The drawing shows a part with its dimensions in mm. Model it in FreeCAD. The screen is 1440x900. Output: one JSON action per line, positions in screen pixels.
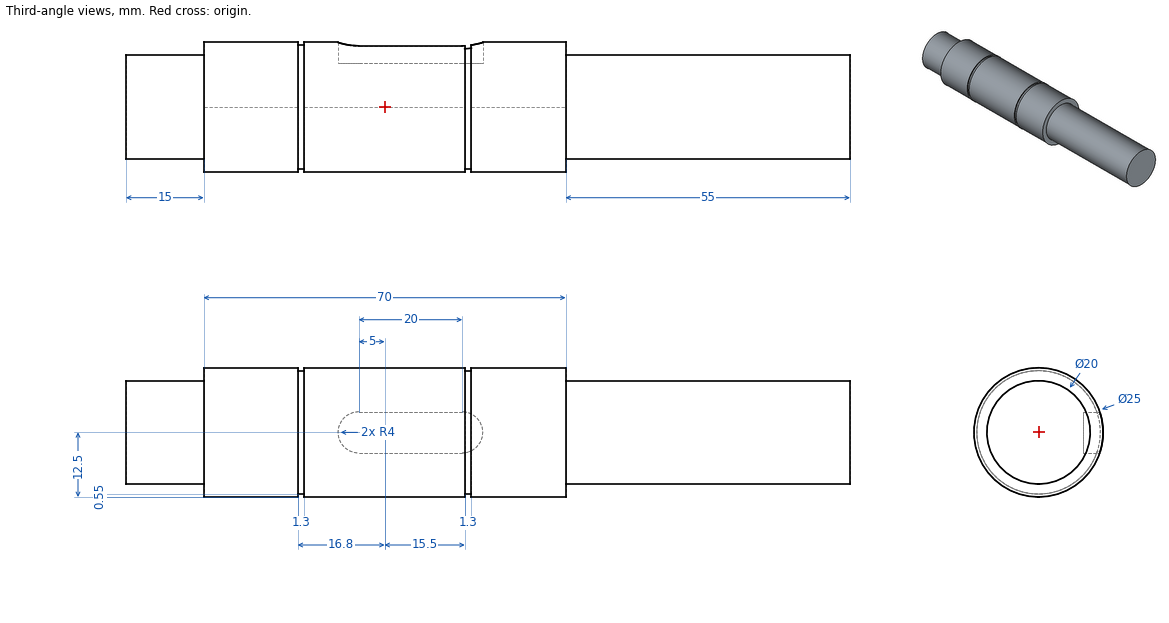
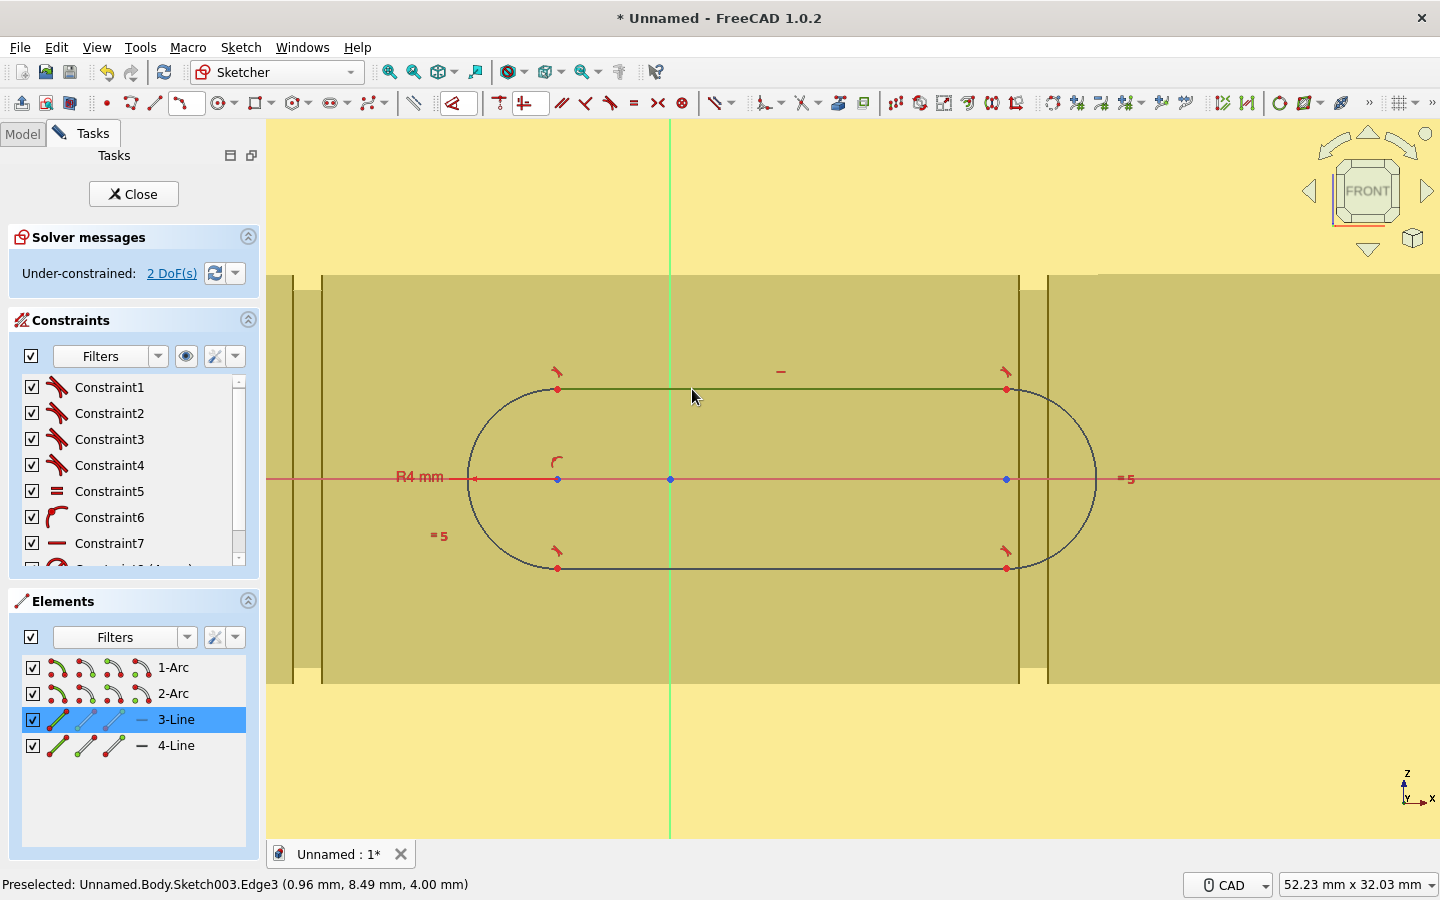
{"action": "key", "text": "l"}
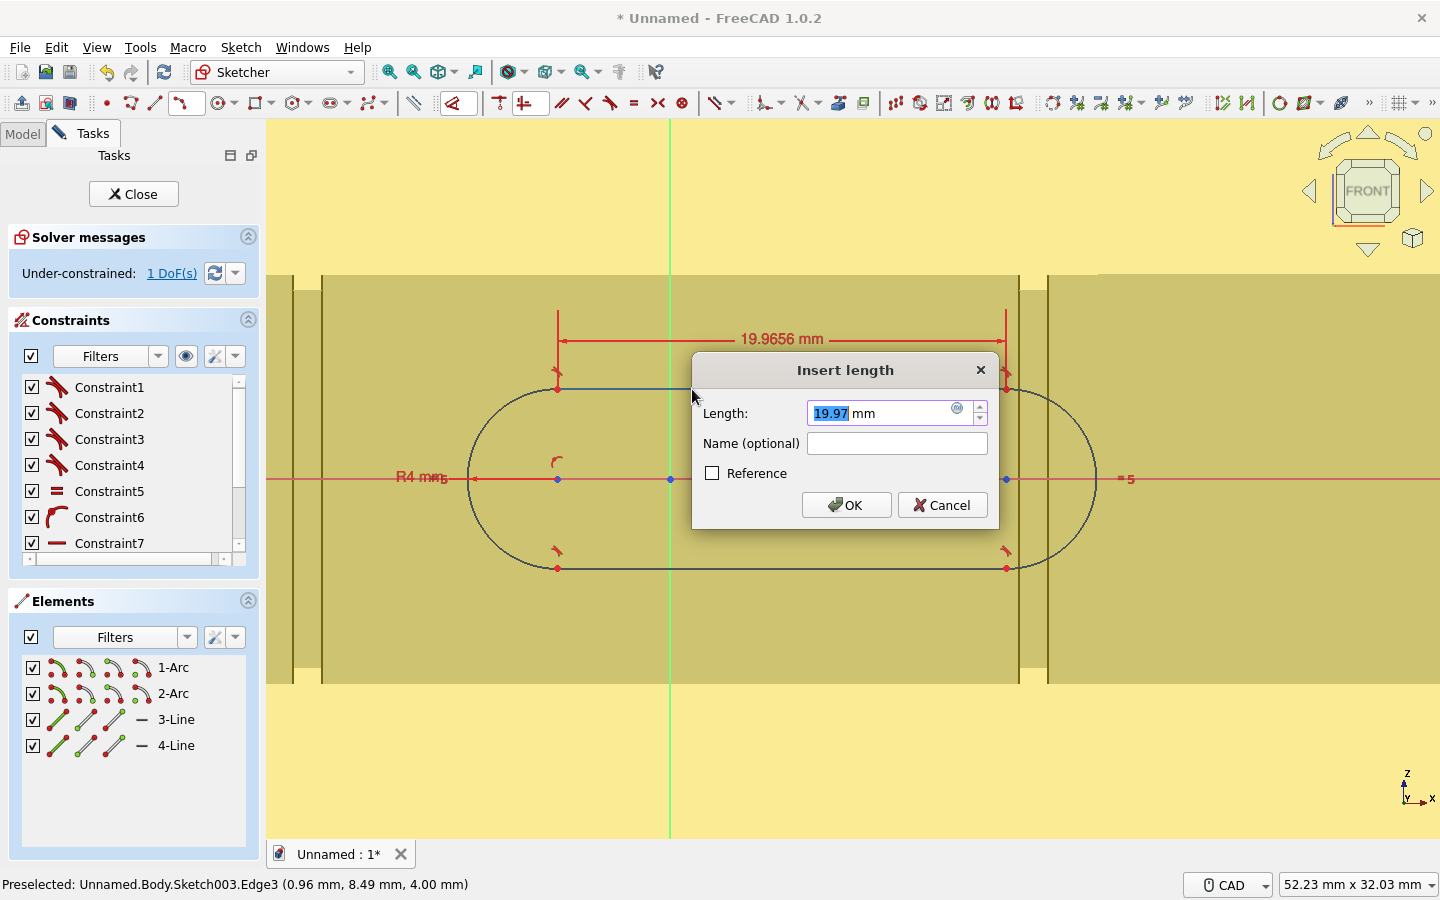
{"action": "type", "text": "20"}
{"action": "key", "text": "Return"}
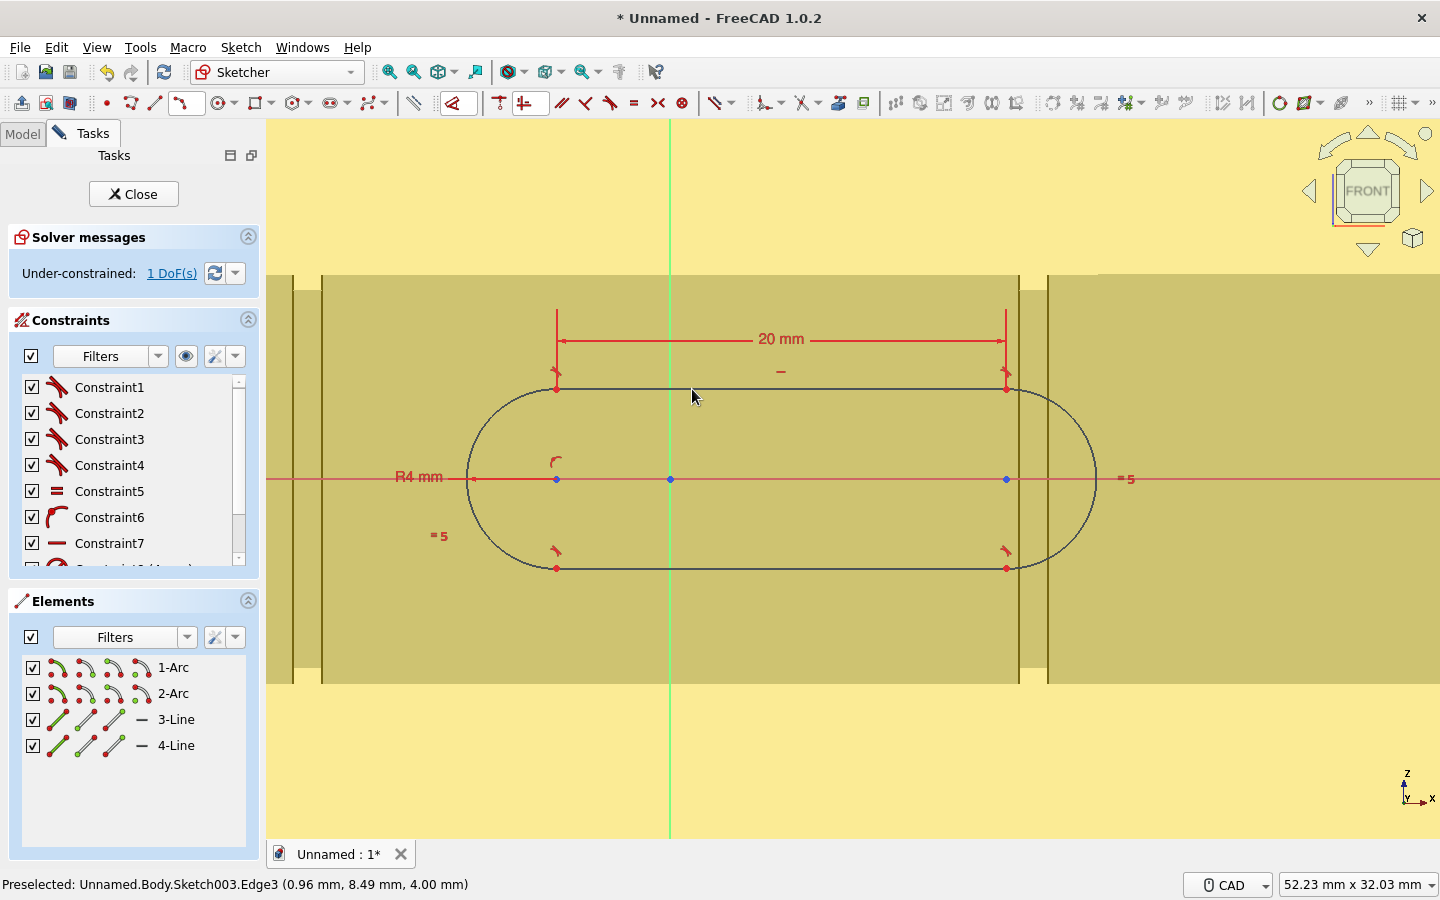
{"action": "left_click", "coordinate": [557, 389]}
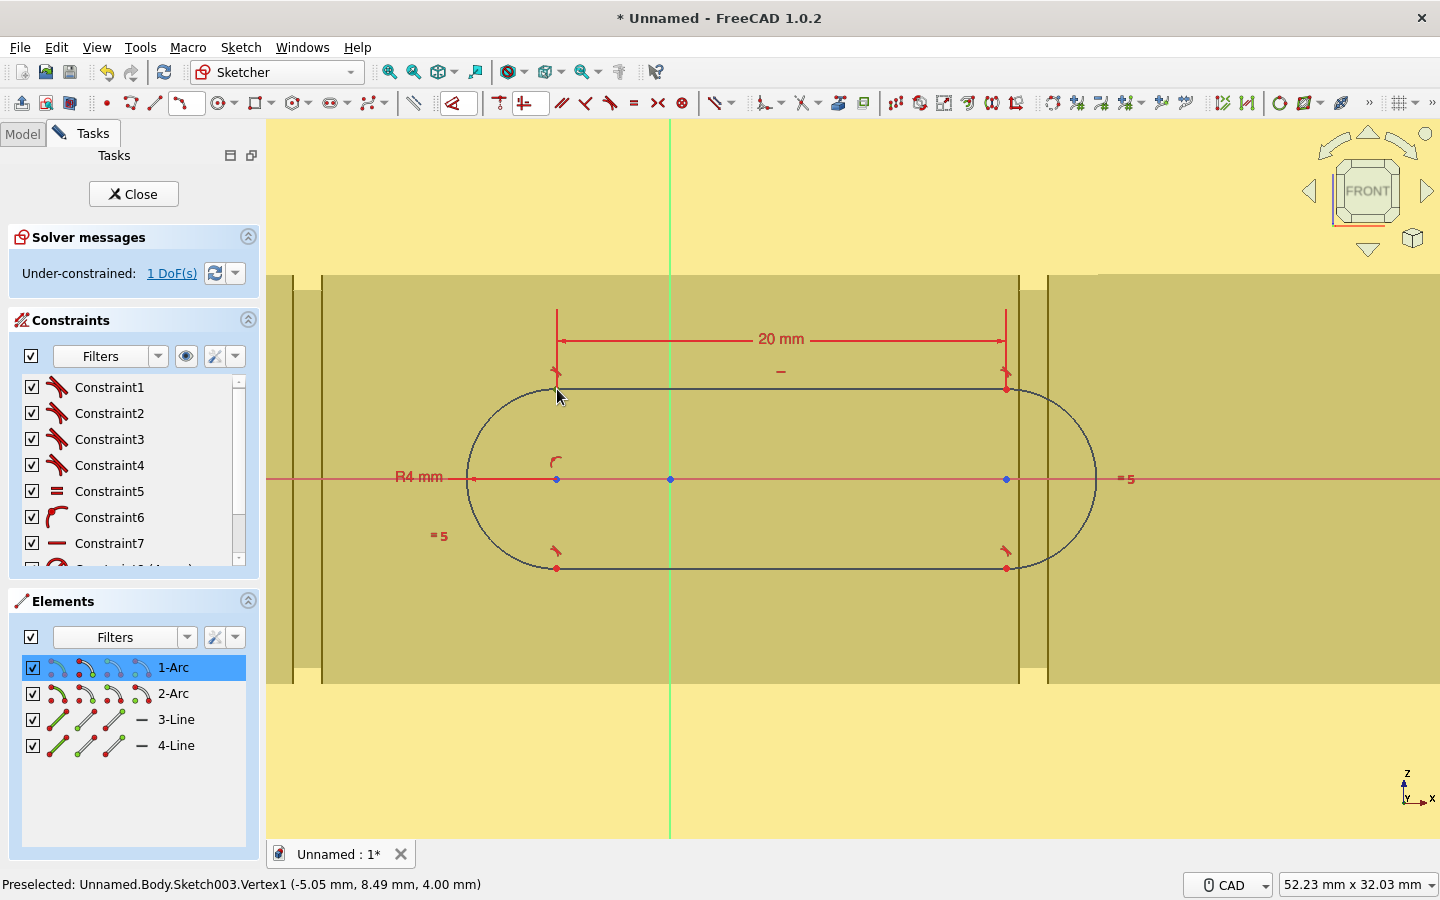
{"action": "left_click", "coordinate": [472, 104]}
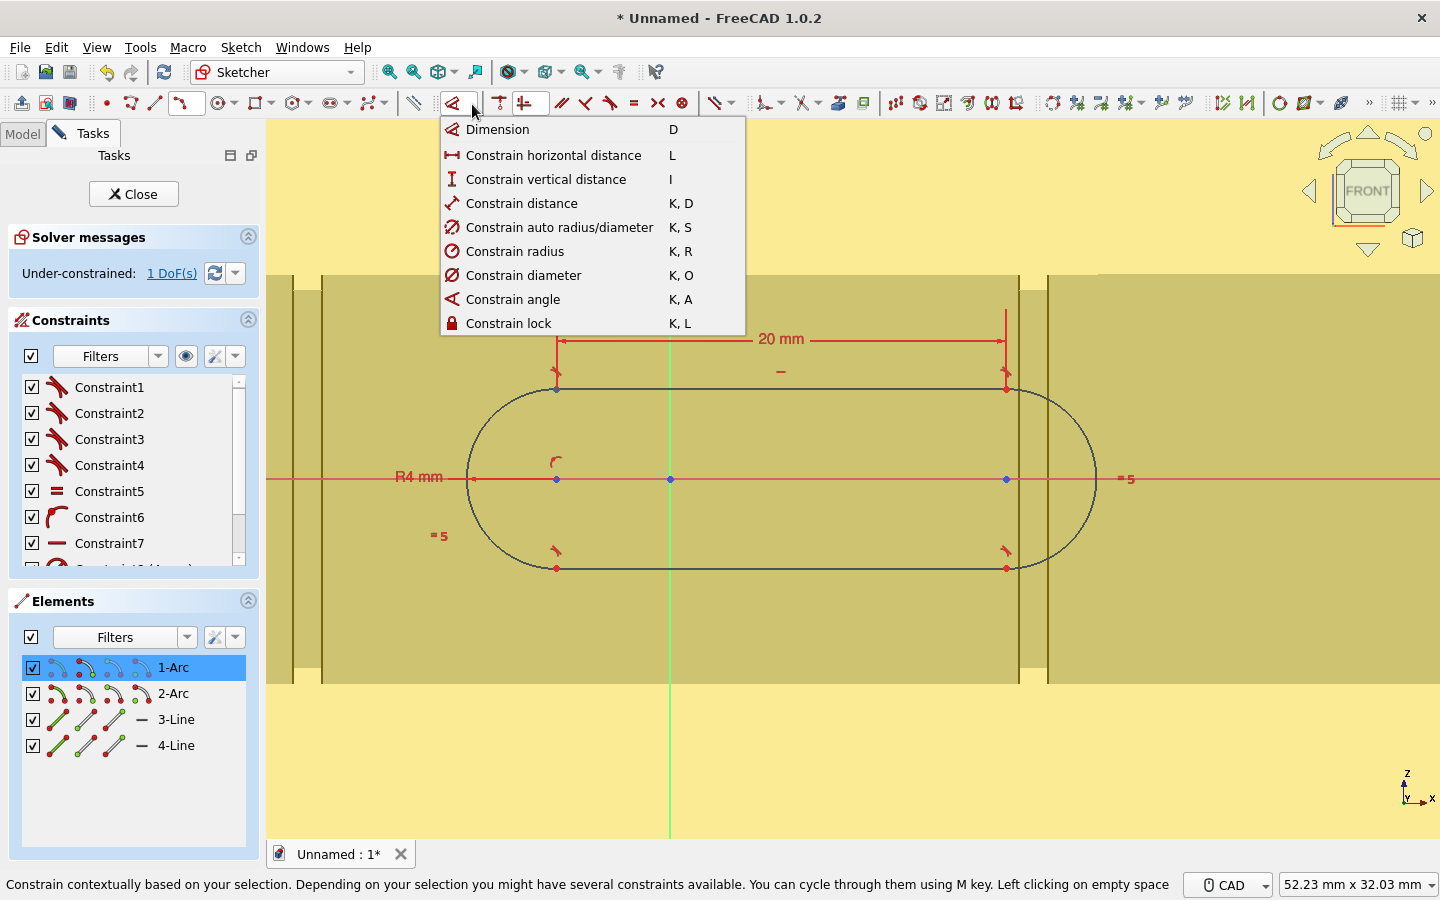
{"action": "left_click", "coordinate": [593, 155]}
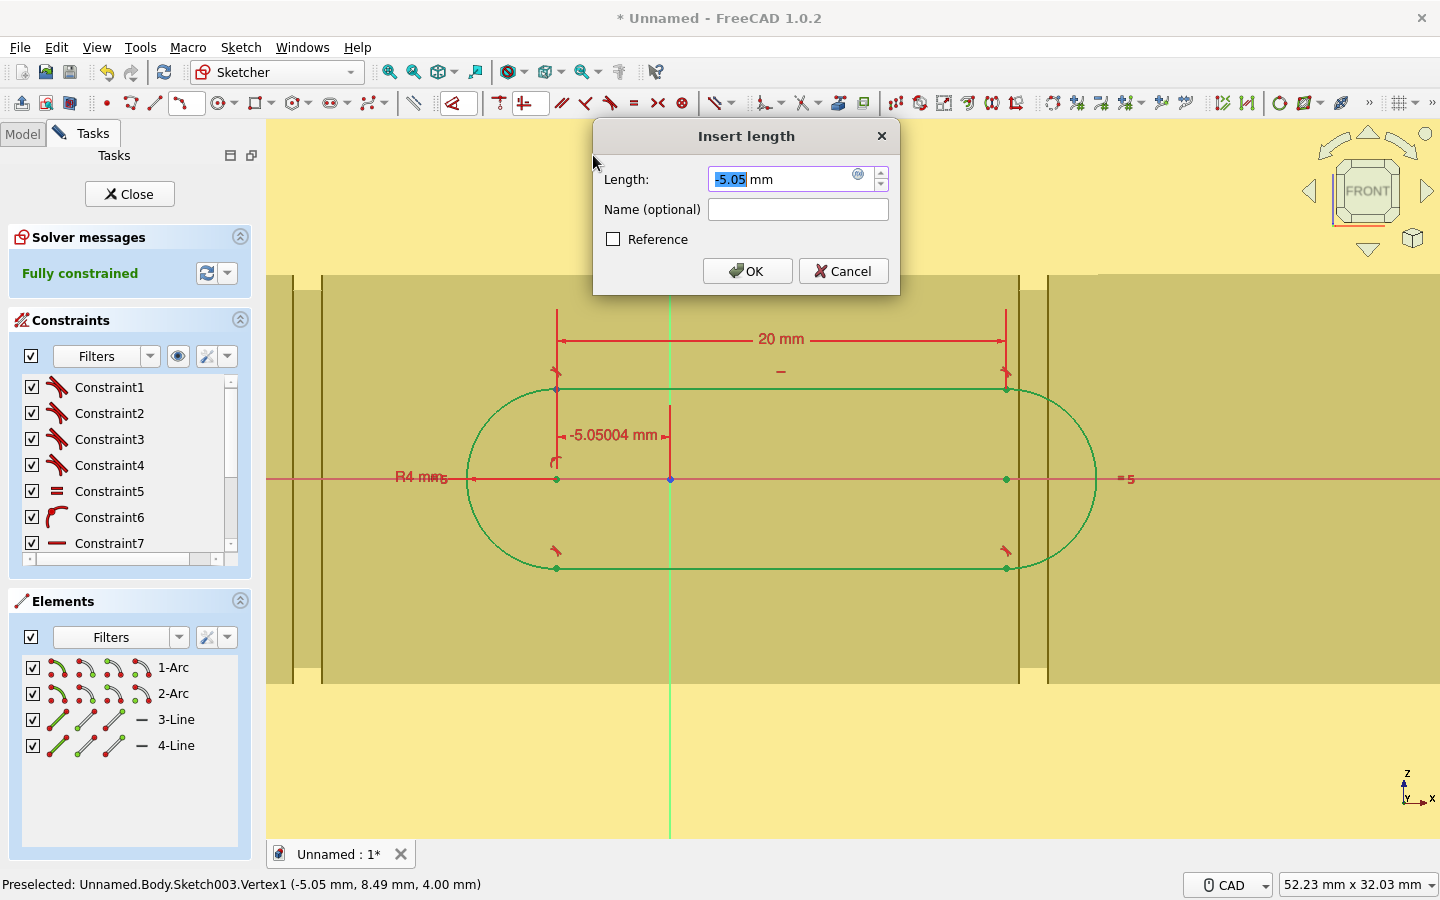
{"action": "type", "text": "-5"}
{"action": "key", "text": "Return"}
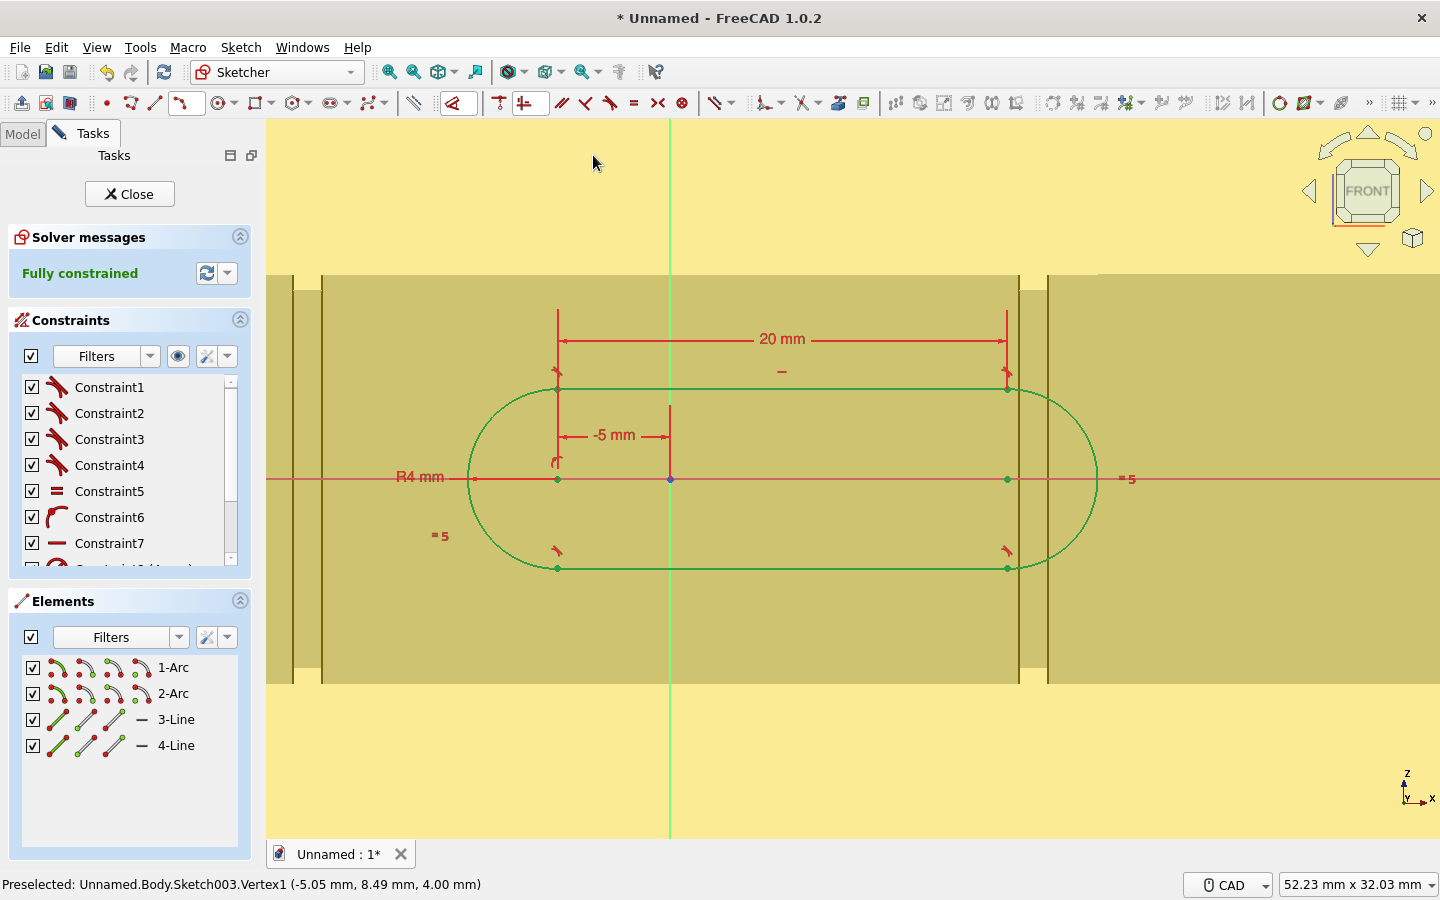
{"action": "left_click", "coordinate": [130, 194]}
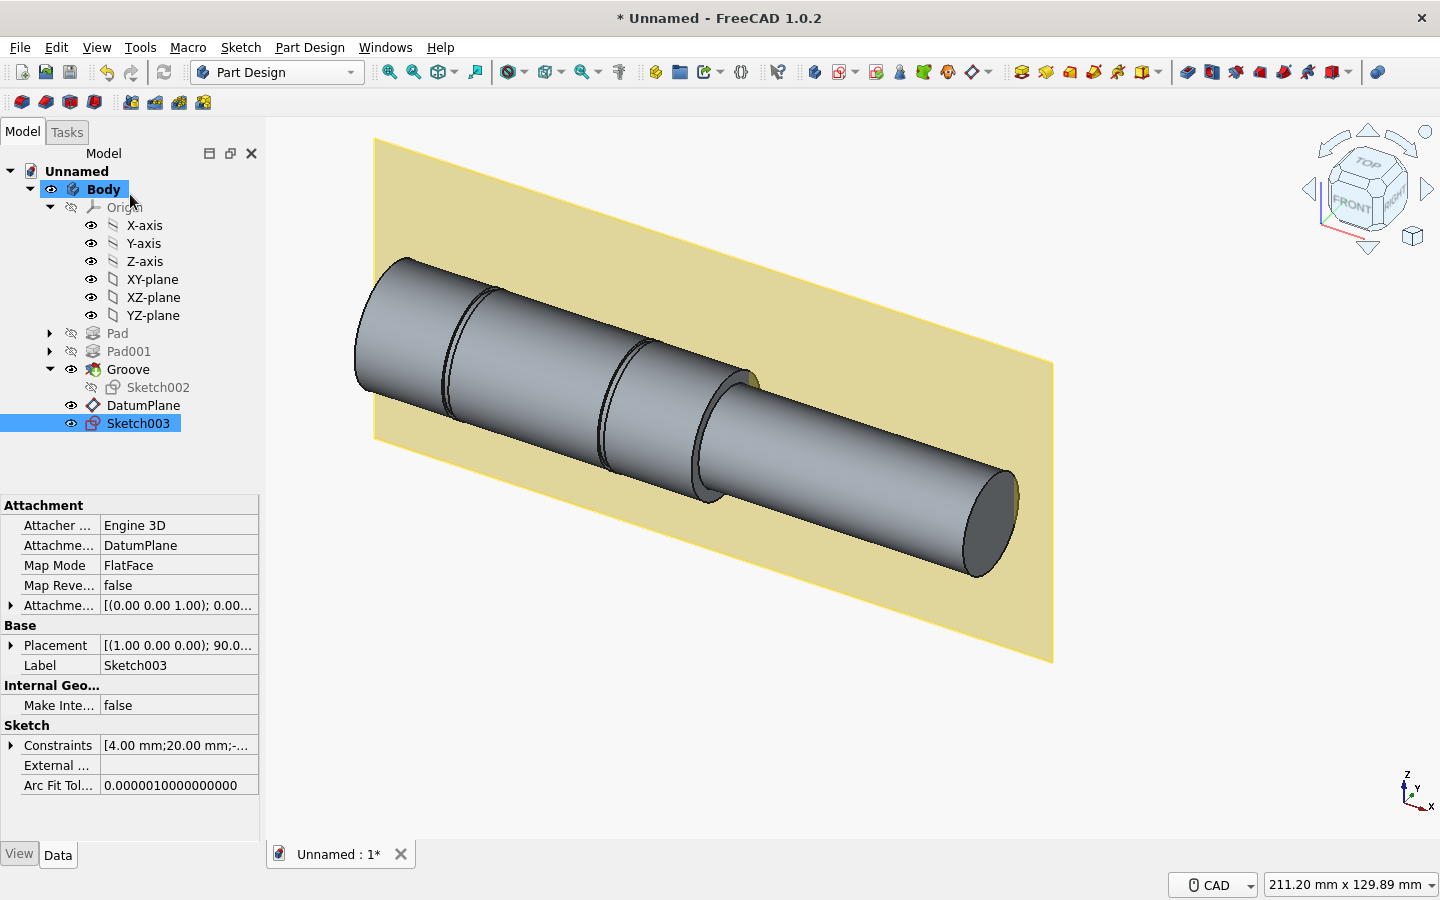
{"action": "left_click", "coordinate": [1188, 72]}